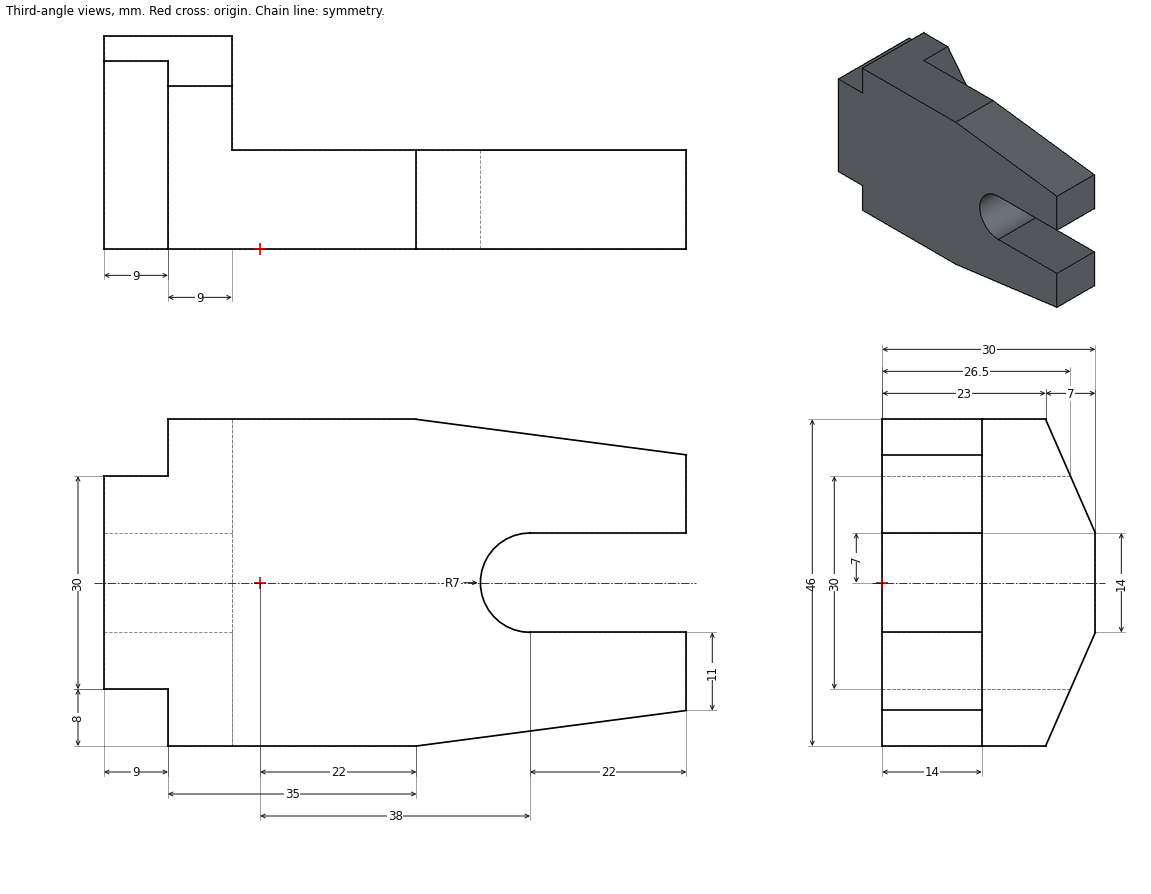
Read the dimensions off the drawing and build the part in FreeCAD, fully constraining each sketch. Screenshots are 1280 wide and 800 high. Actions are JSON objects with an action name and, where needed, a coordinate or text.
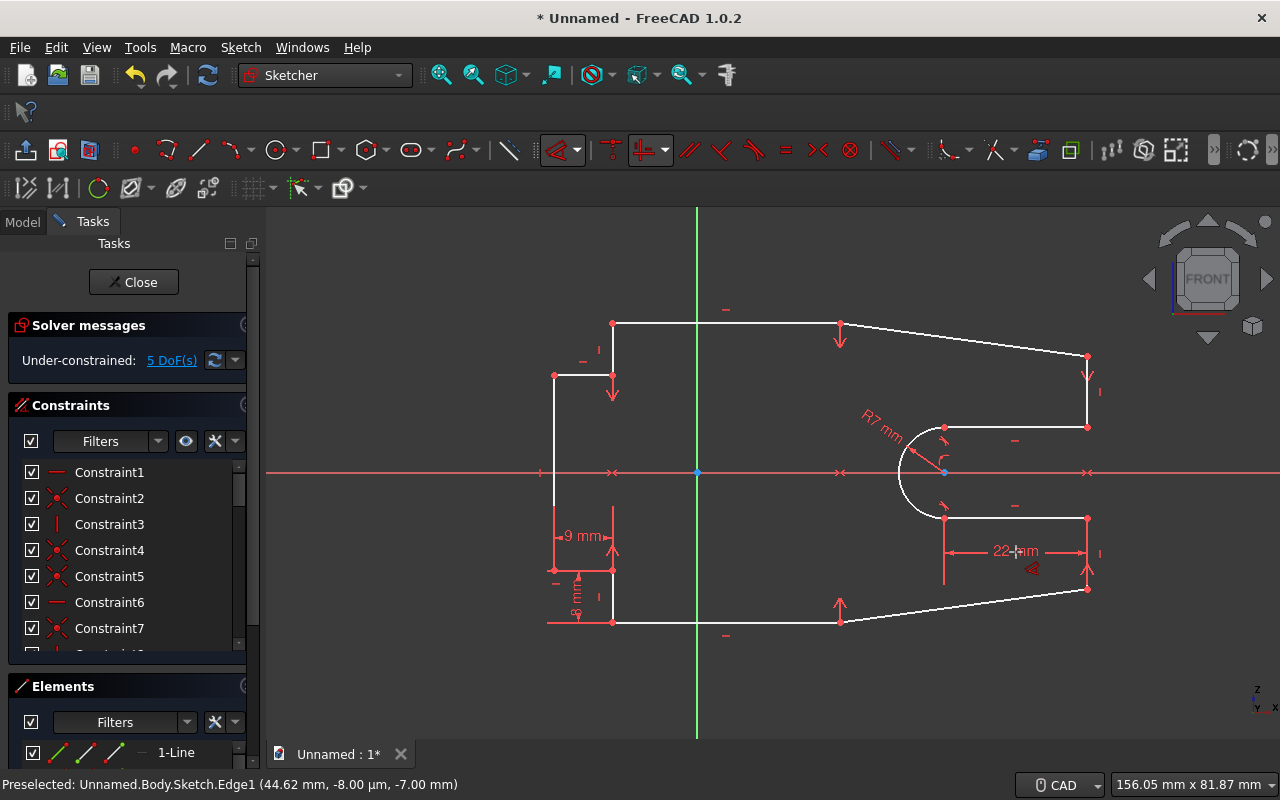
{"action": "left_click", "coordinate": [1087, 540]}
{"action": "left_click", "coordinate": [1053, 579]}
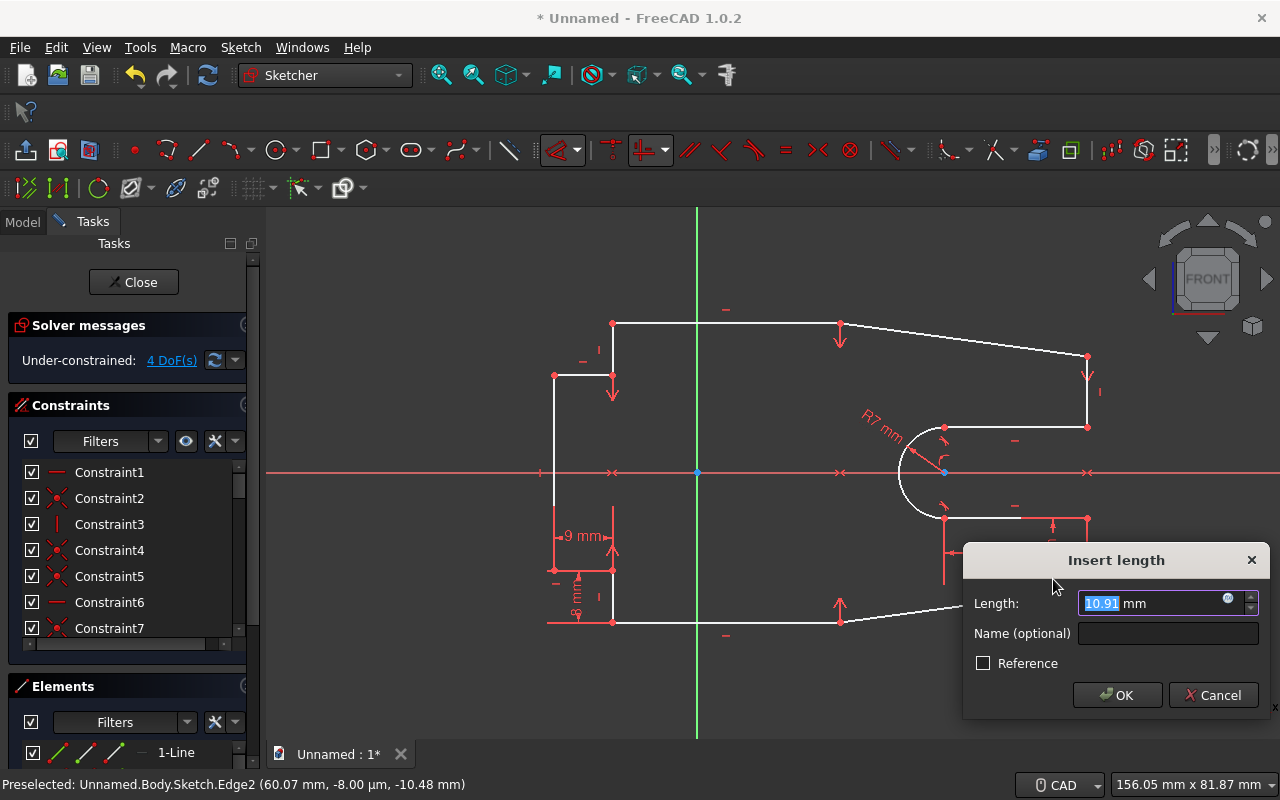
{"action": "type", "text": "11"}
{"action": "key", "text": "Return"}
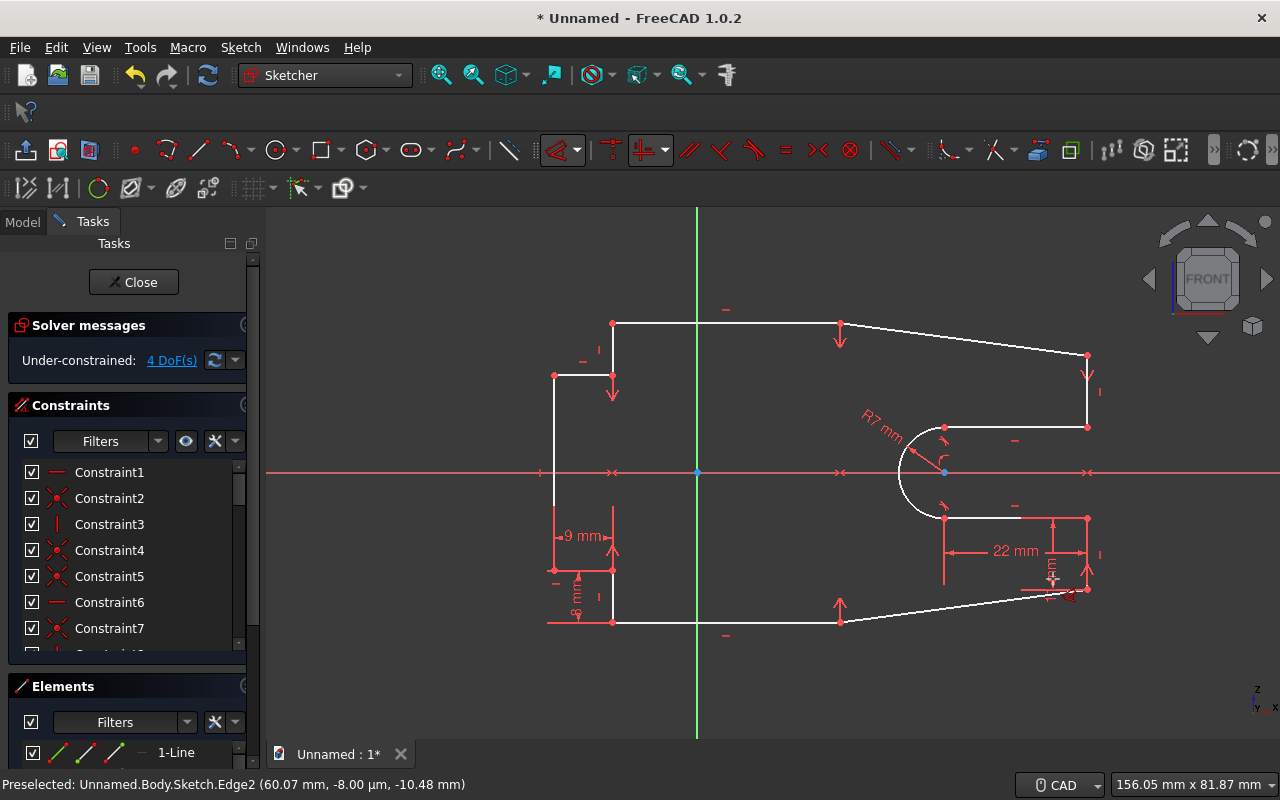
{"action": "left_click", "coordinate": [772, 623]}
{"action": "left_click", "coordinate": [726, 657]}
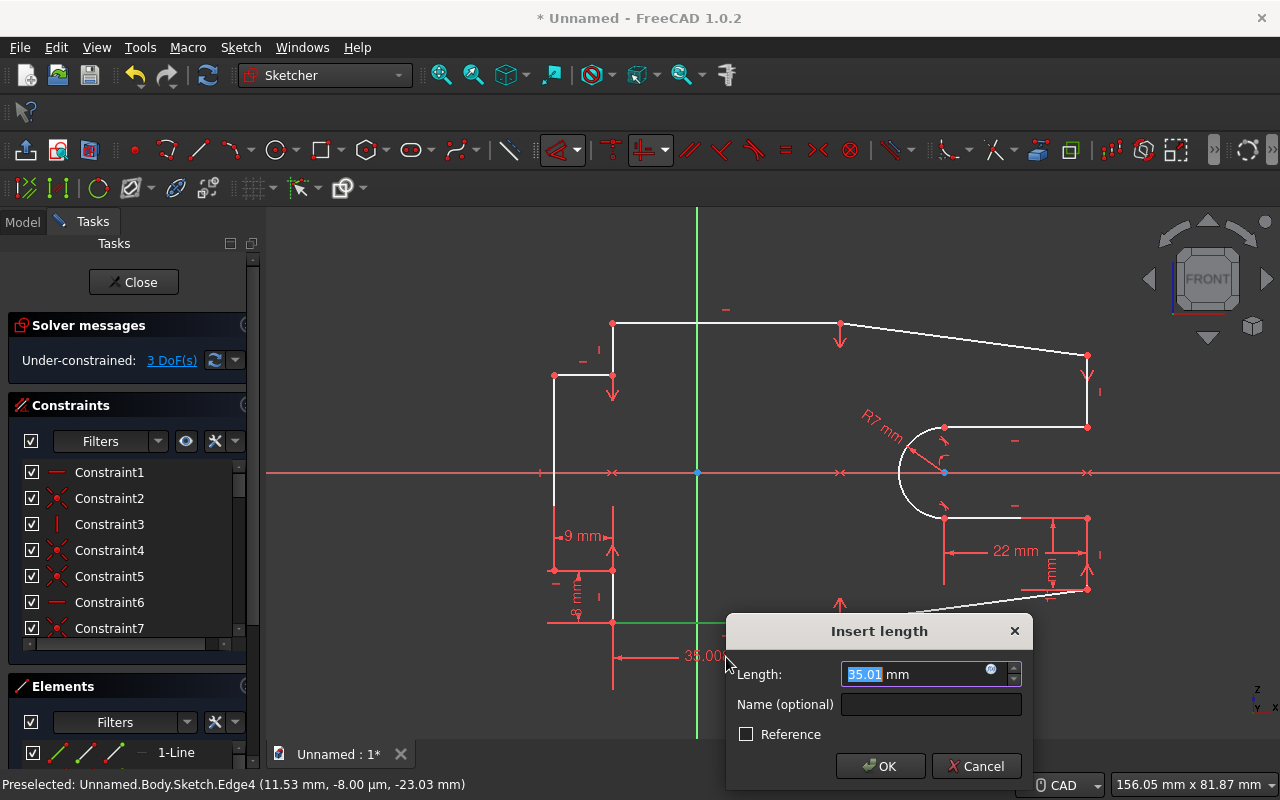
{"action": "type", "text": "35"}
{"action": "key", "text": "Return"}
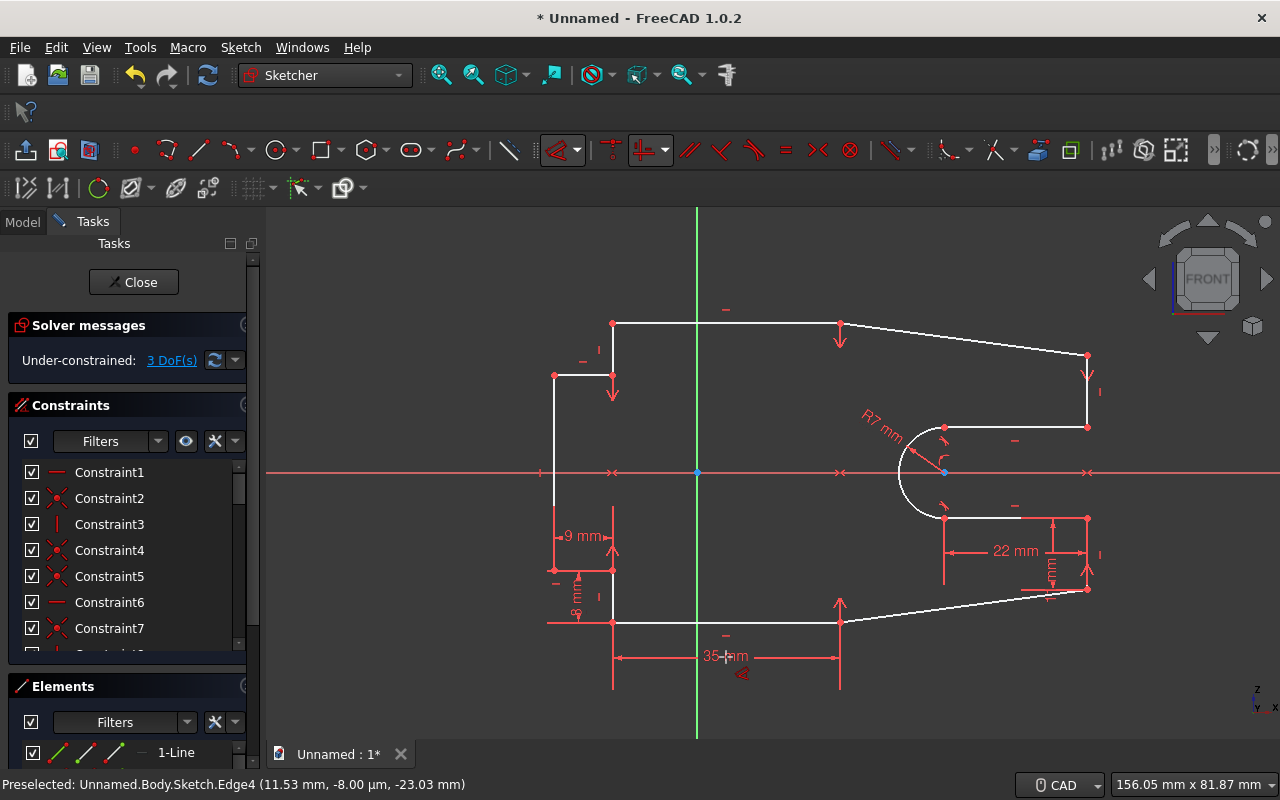
{"action": "left_click", "coordinate": [554, 512]}
{"action": "left_click", "coordinate": [520, 428]}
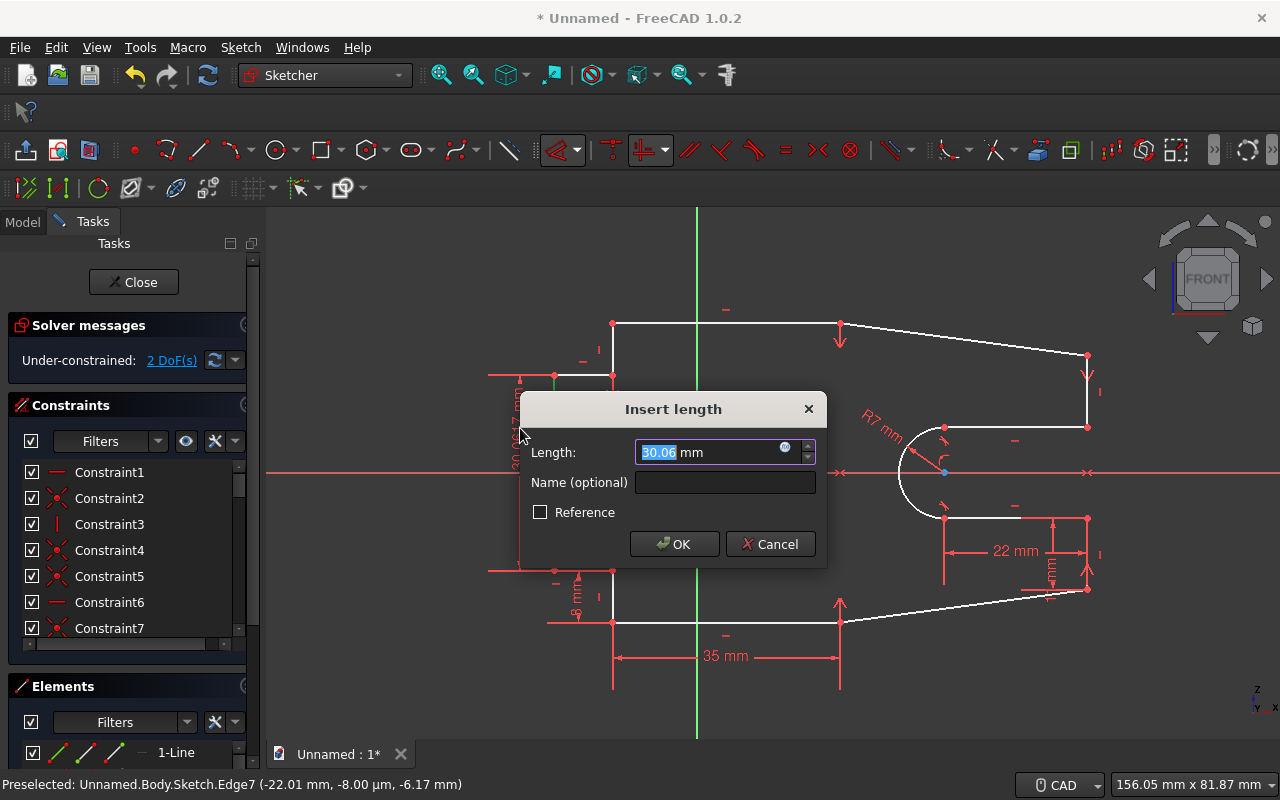
{"action": "type", "text": "30"}
{"action": "key", "text": "Return"}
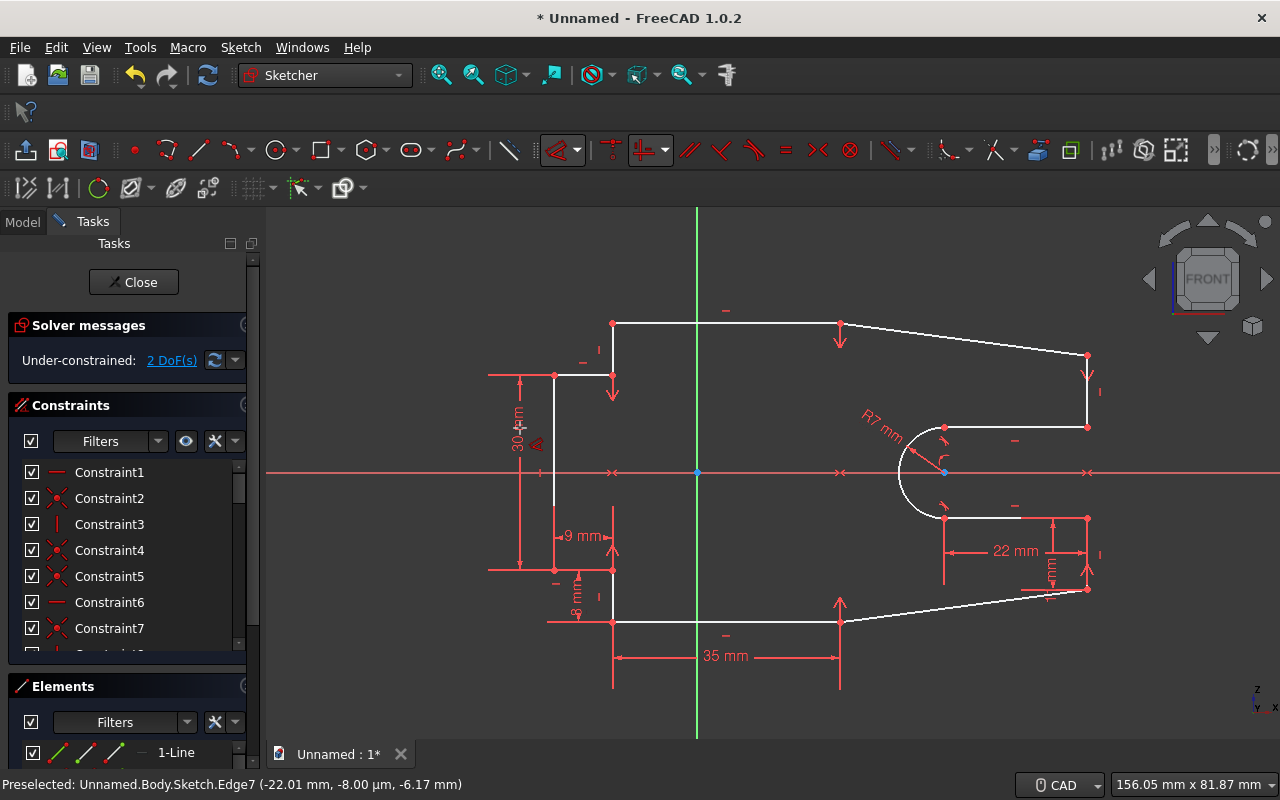
{"action": "left_click", "coordinate": [944, 518]}
{"action": "left_click", "coordinate": [821, 552]}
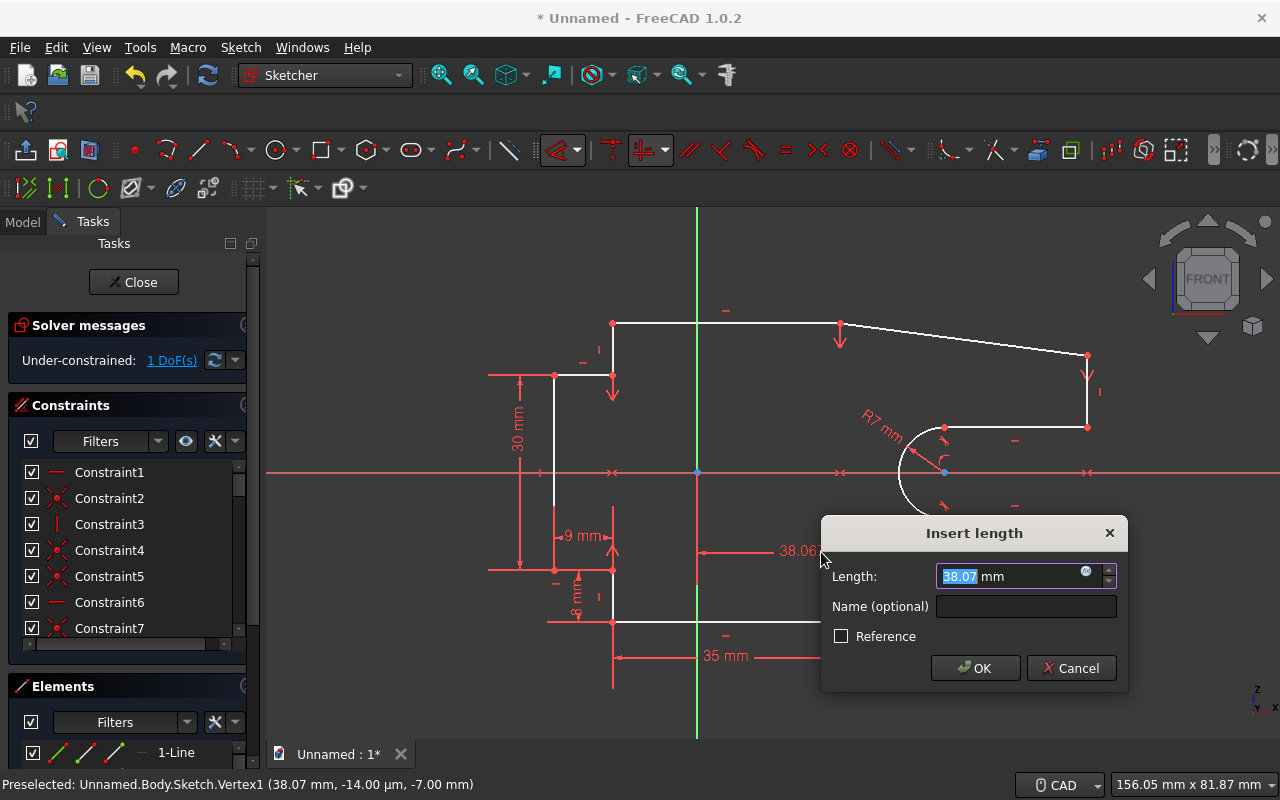
{"action": "type", "text": "38"}
{"action": "key", "text": "Return"}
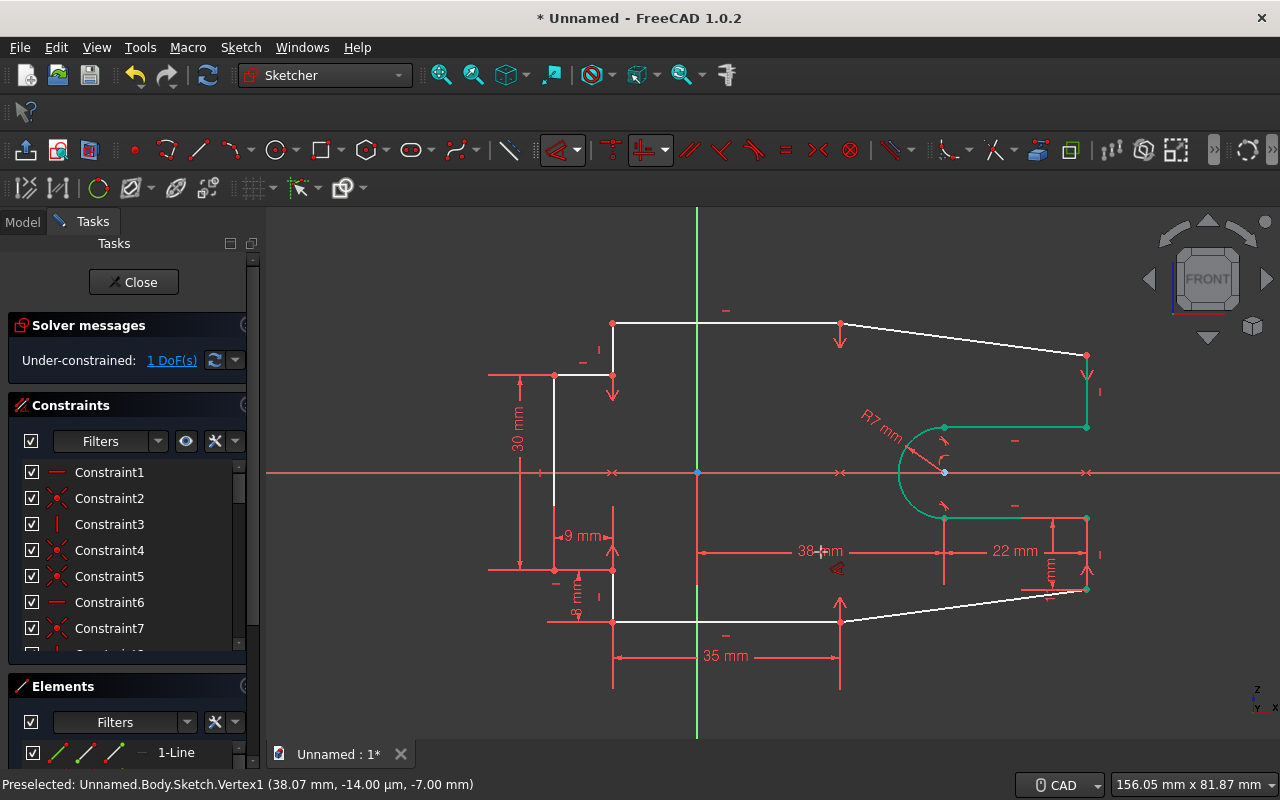
{"action": "left_click", "coordinate": [840, 622]}
{"action": "left_click", "coordinate": [801, 656]}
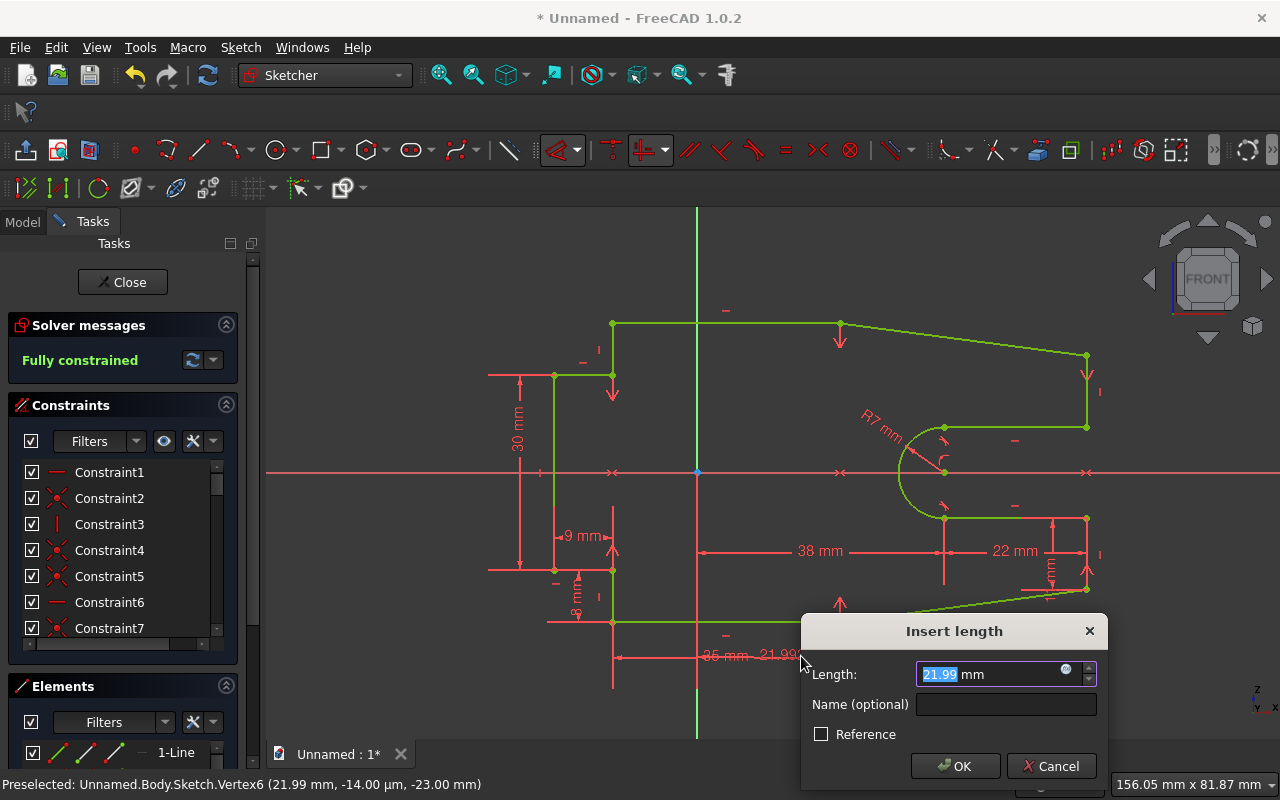
{"action": "type", "text": "22"}
{"action": "key", "text": "Return"}
{"action": "key", "text": "Escape"}